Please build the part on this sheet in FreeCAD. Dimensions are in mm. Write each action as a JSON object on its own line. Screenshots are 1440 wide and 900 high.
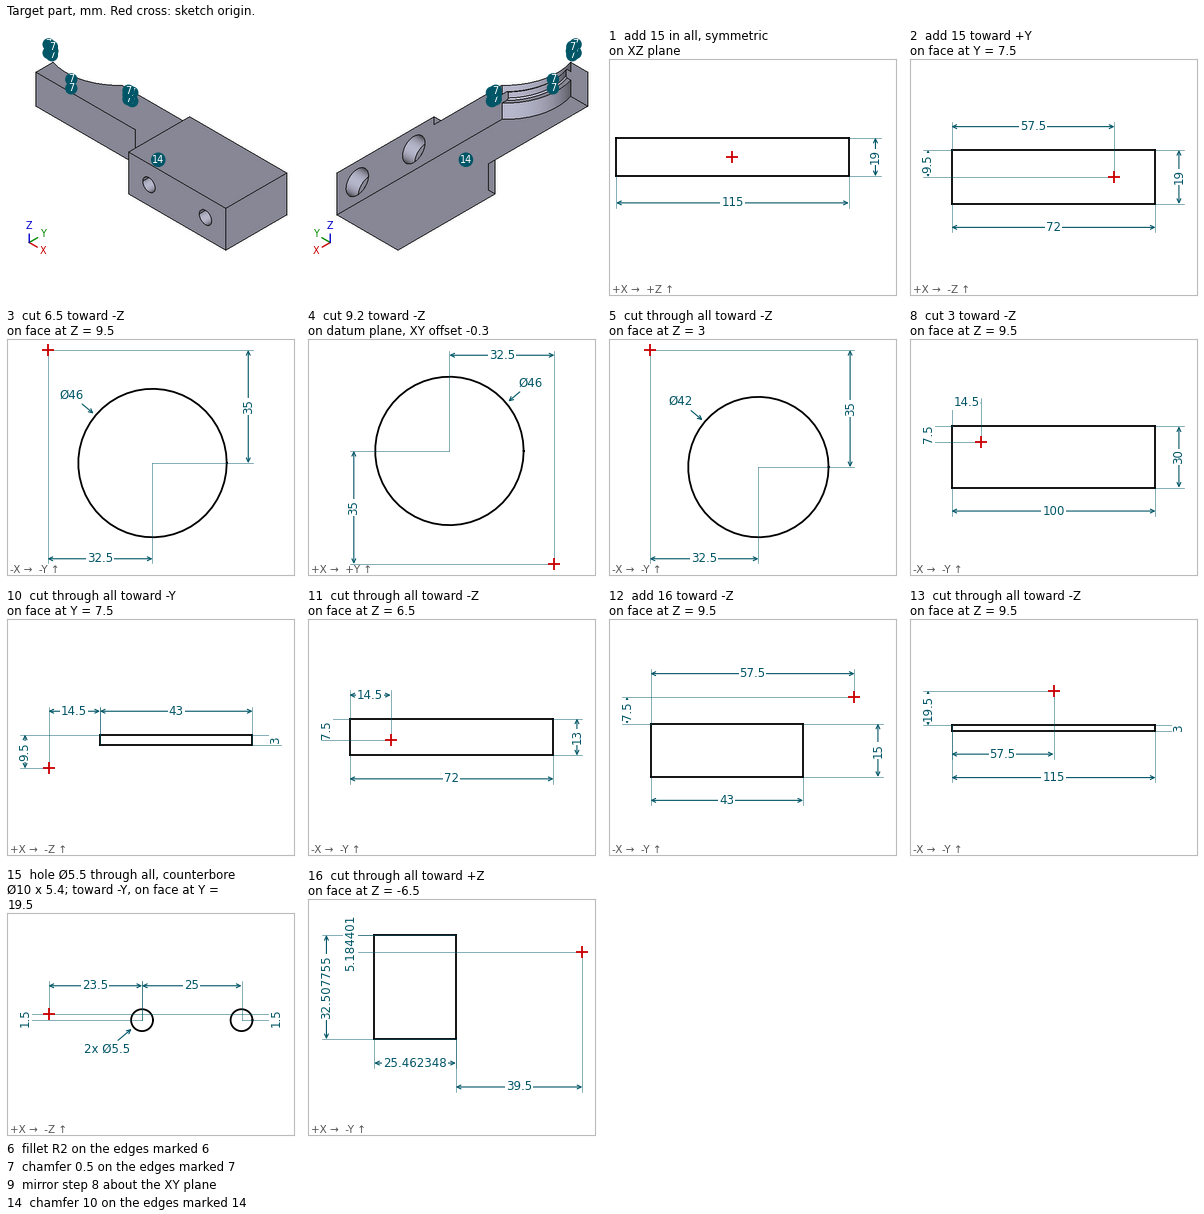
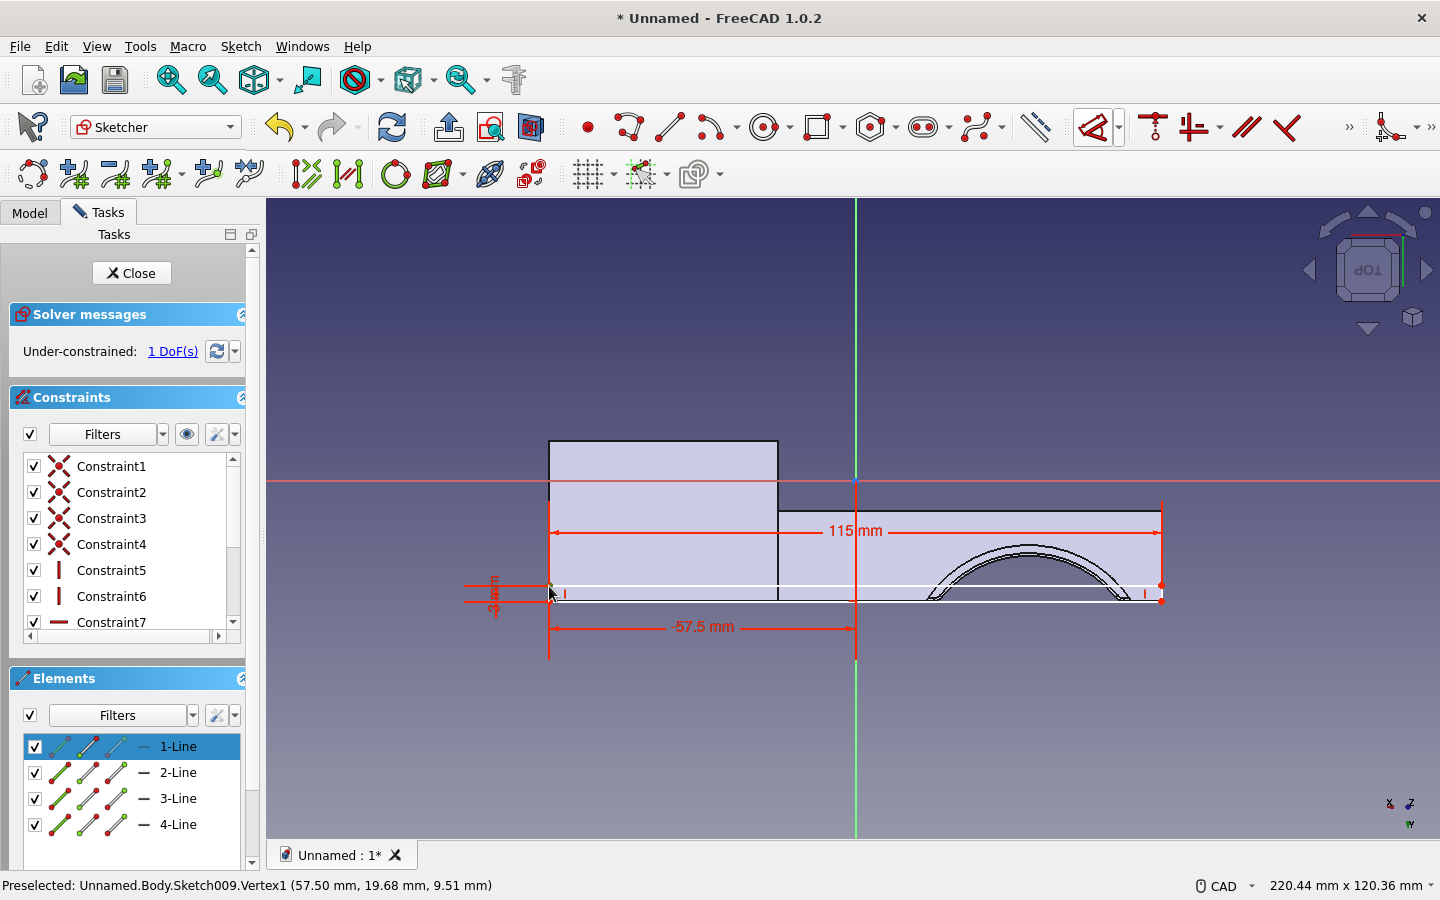
{"action": "left_click", "coordinate": [1118, 128]}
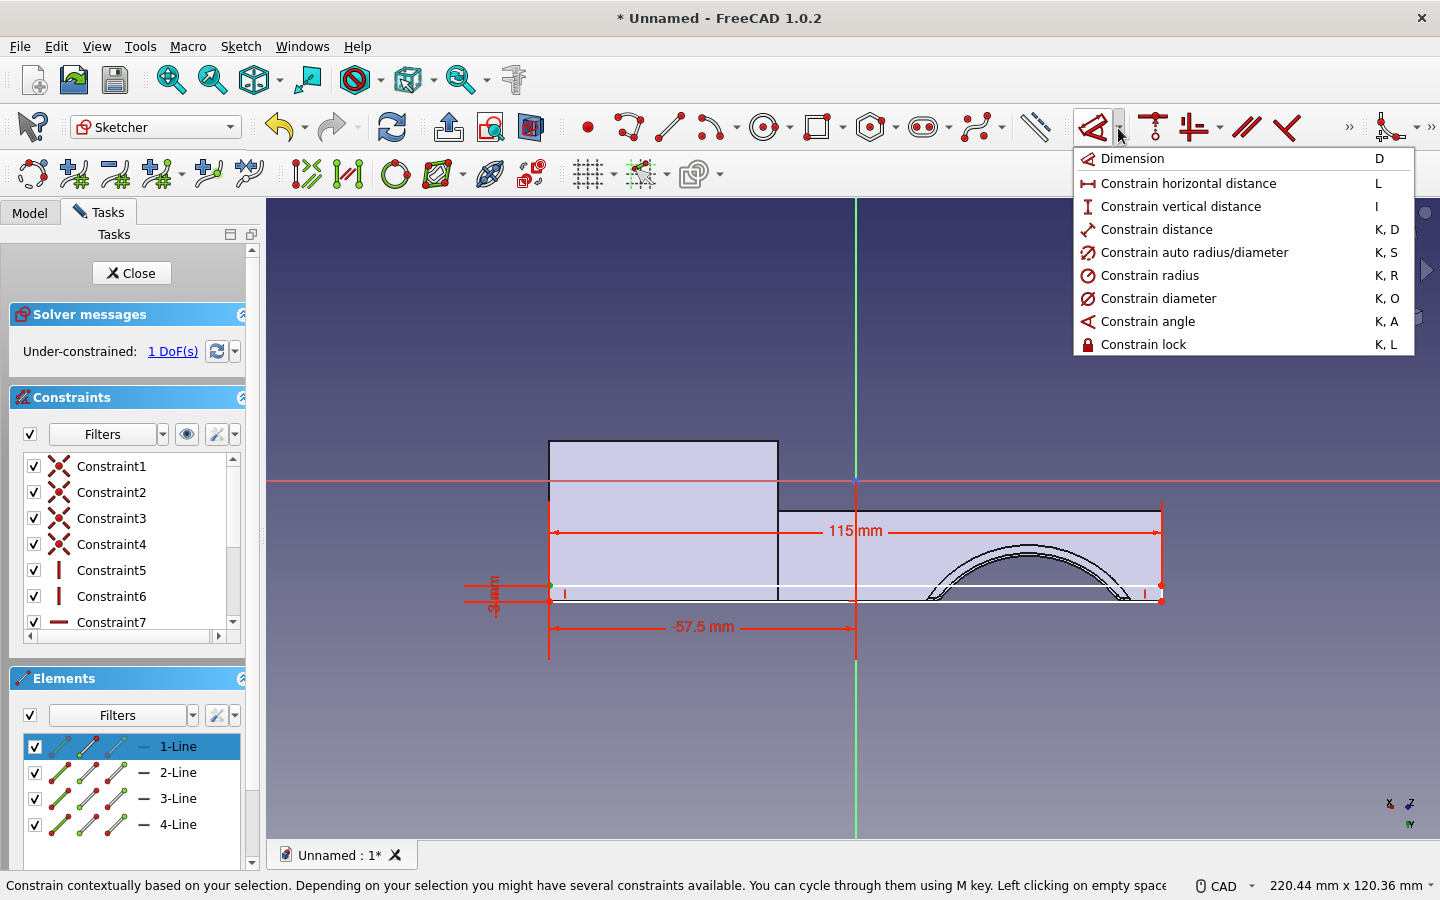
{"action": "left_click", "coordinate": [1244, 206]}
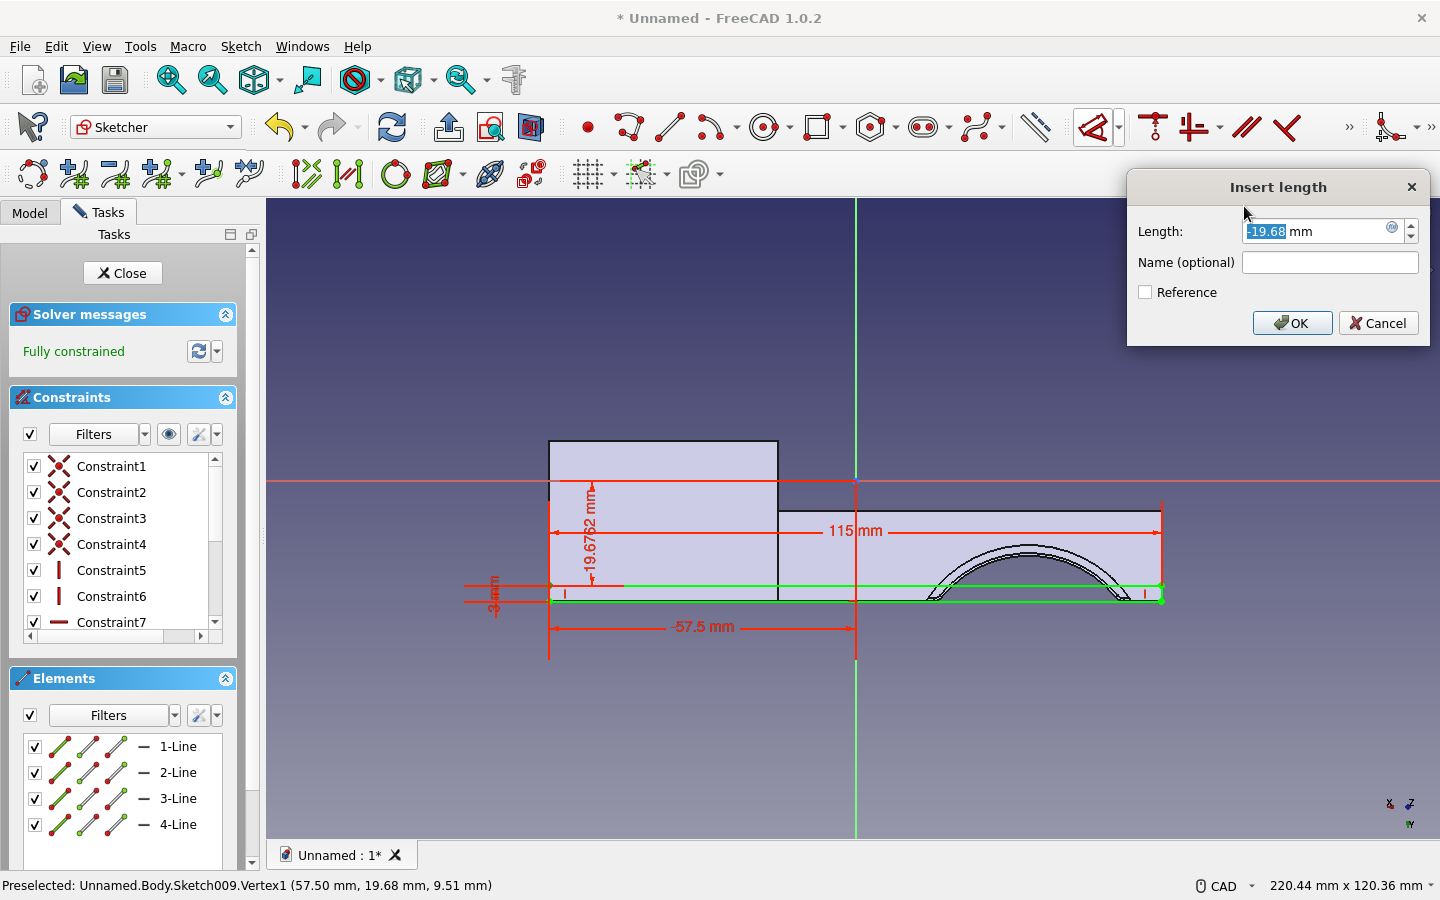
{"action": "type", "text": "-19.5"}
{"action": "key", "text": "Return"}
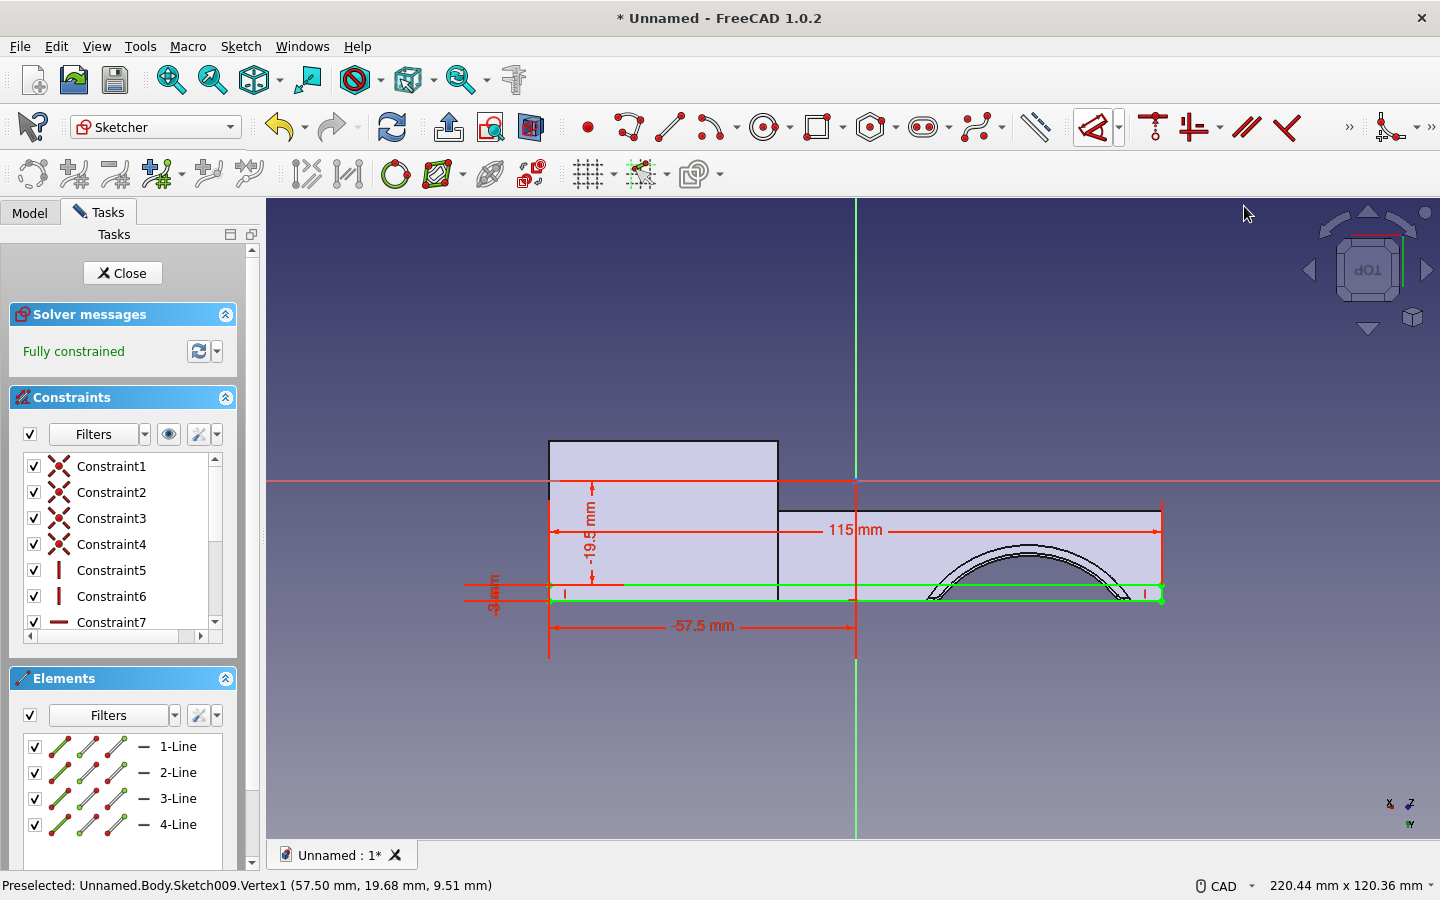
{"action": "left_click", "coordinate": [123, 273]}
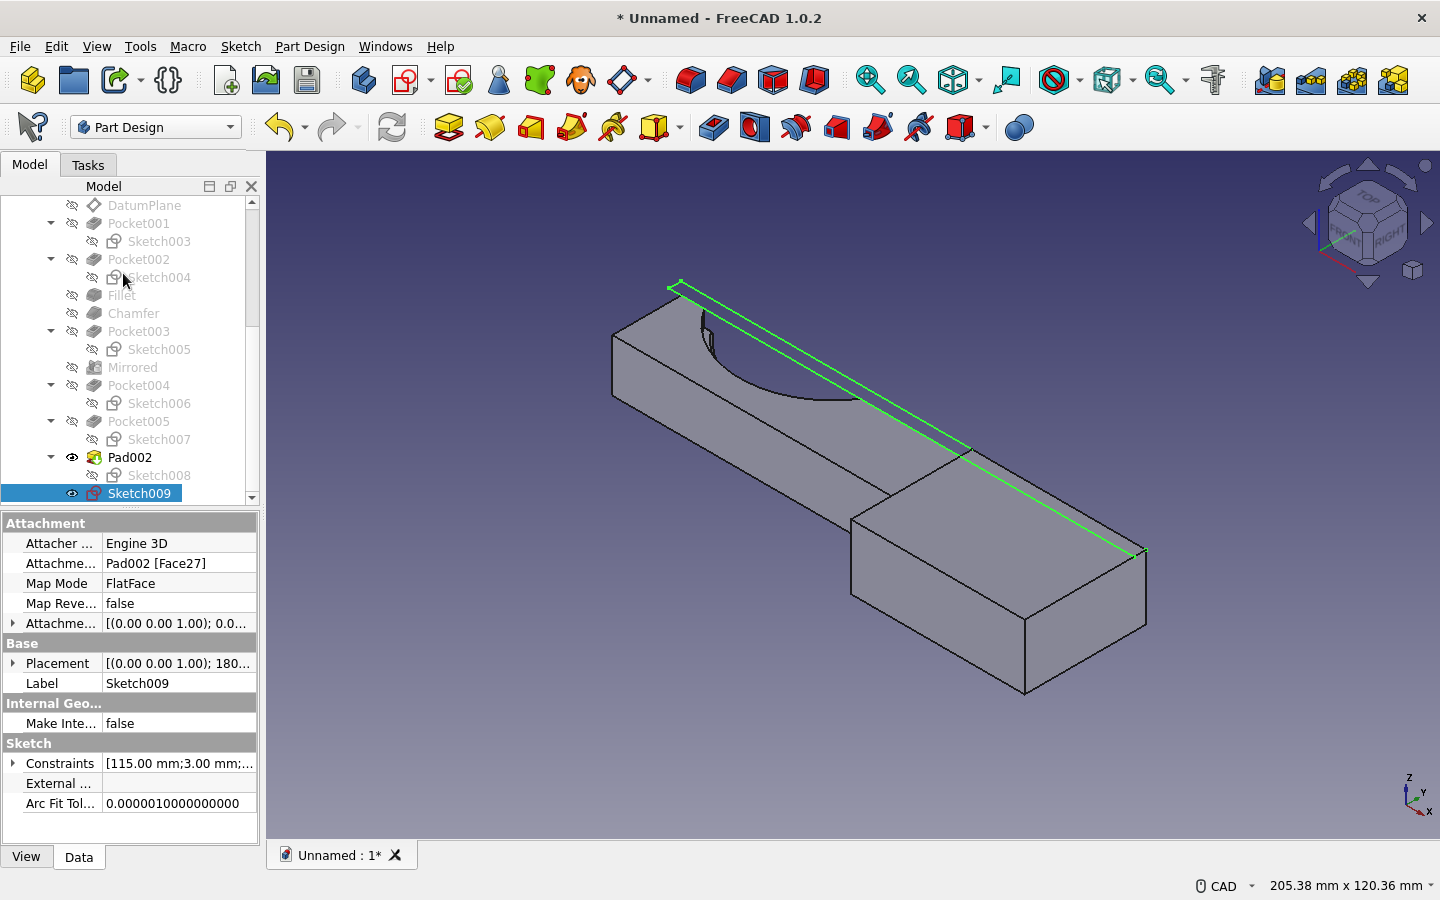
{"action": "left_click", "coordinate": [714, 128]}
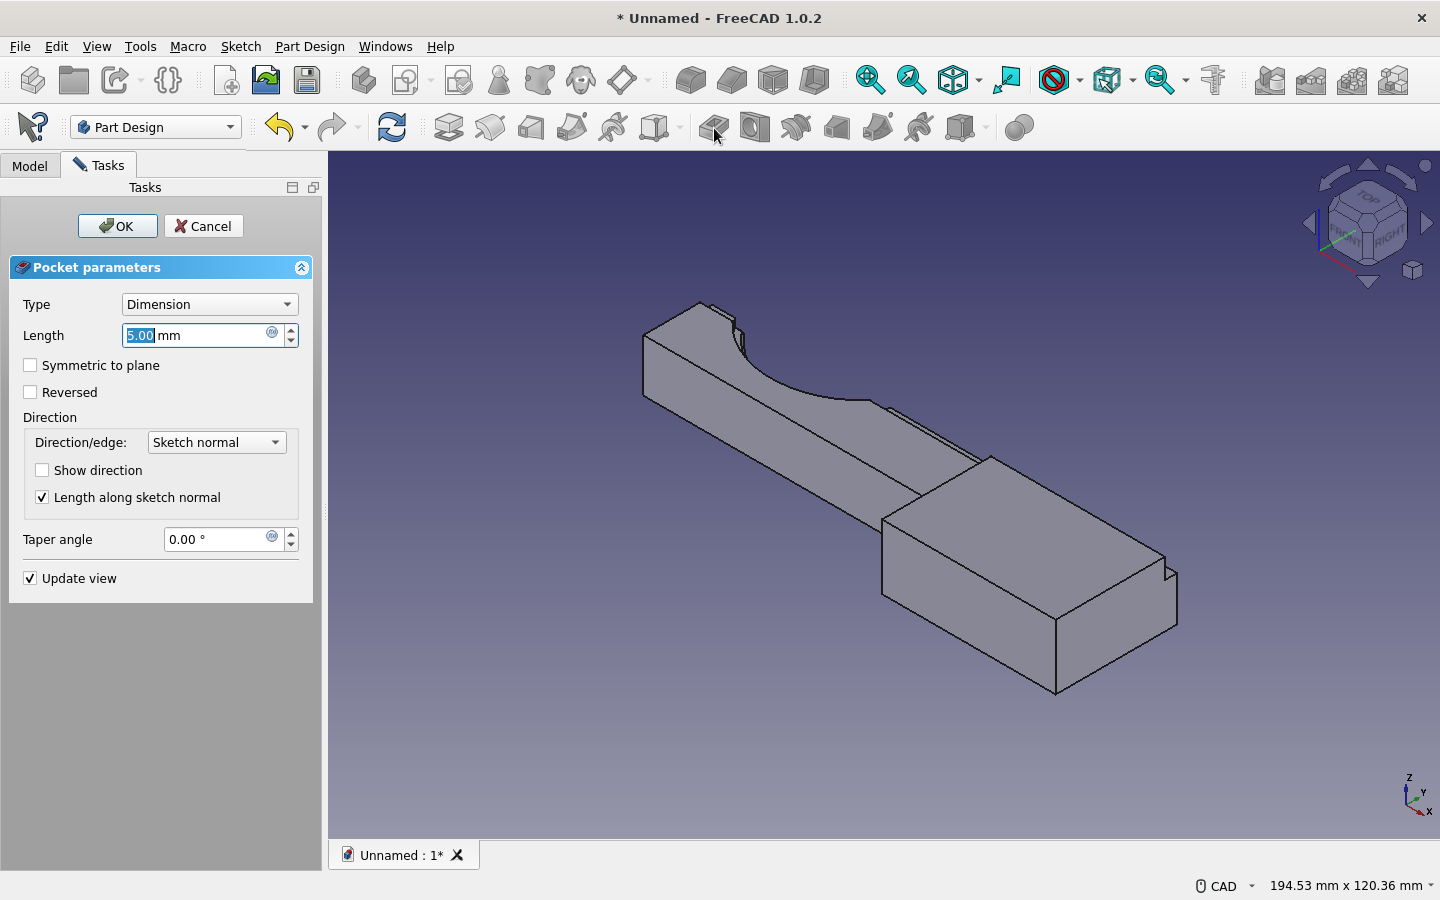
{"action": "left_click", "coordinate": [210, 304]}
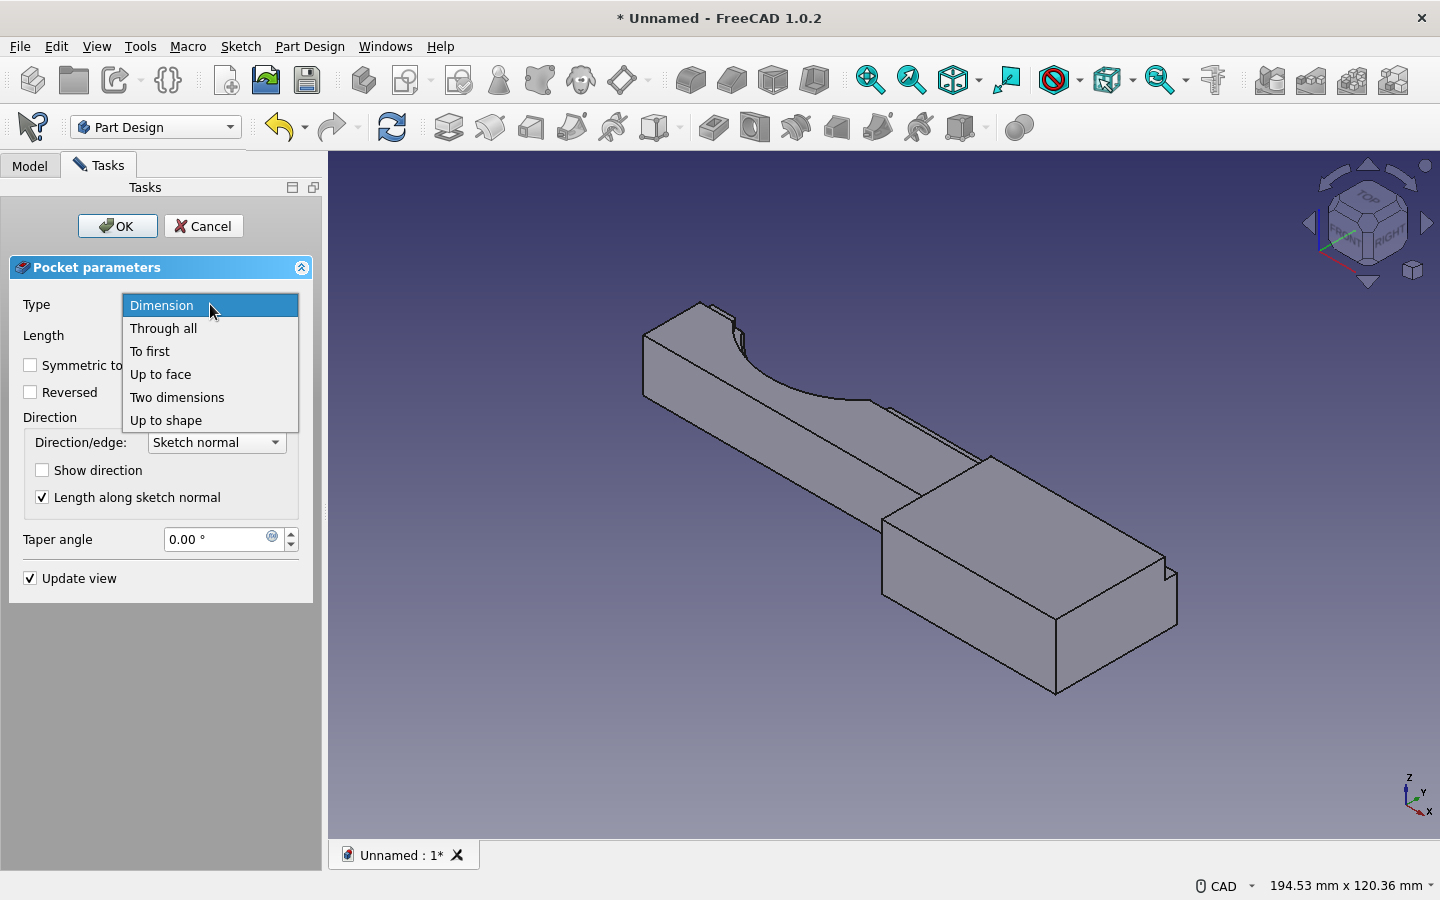
{"action": "left_click", "coordinate": [208, 328]}